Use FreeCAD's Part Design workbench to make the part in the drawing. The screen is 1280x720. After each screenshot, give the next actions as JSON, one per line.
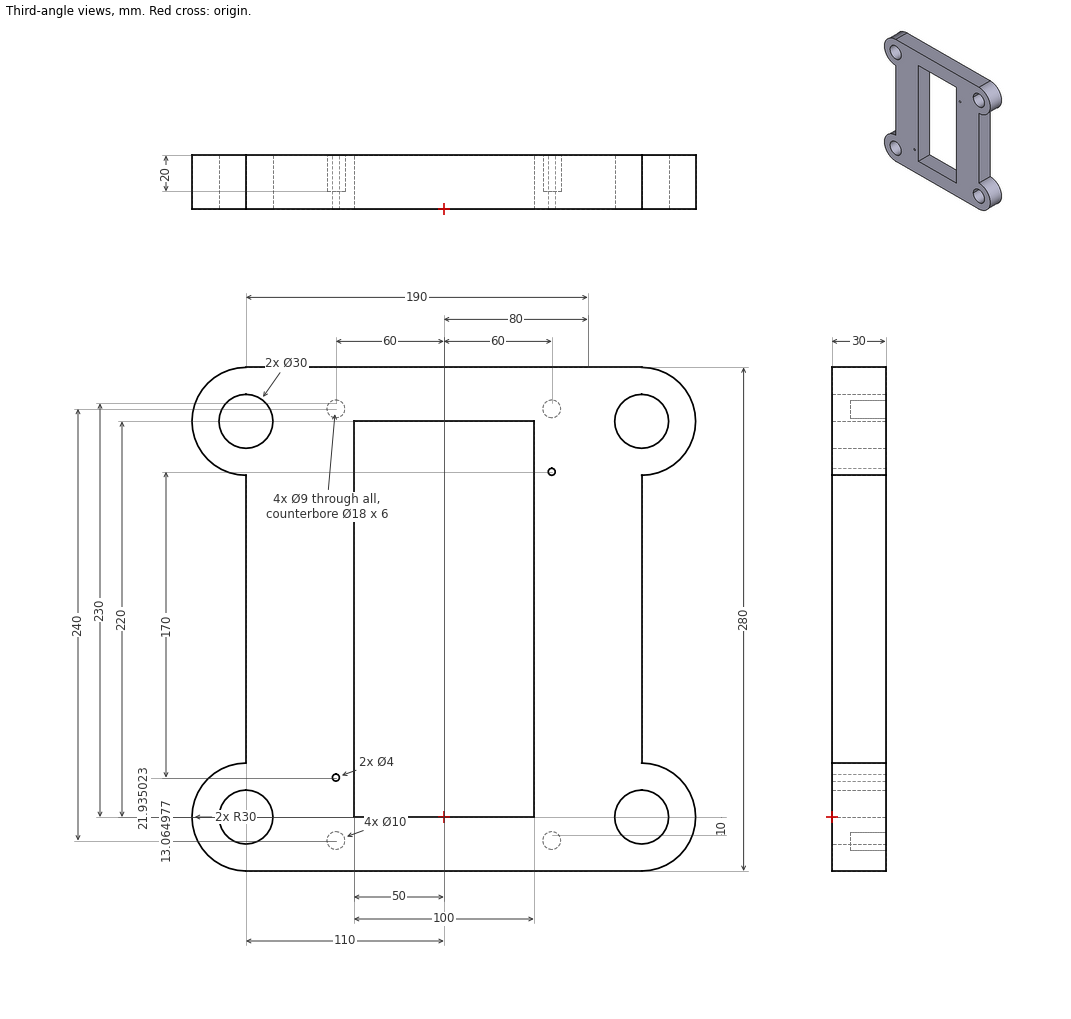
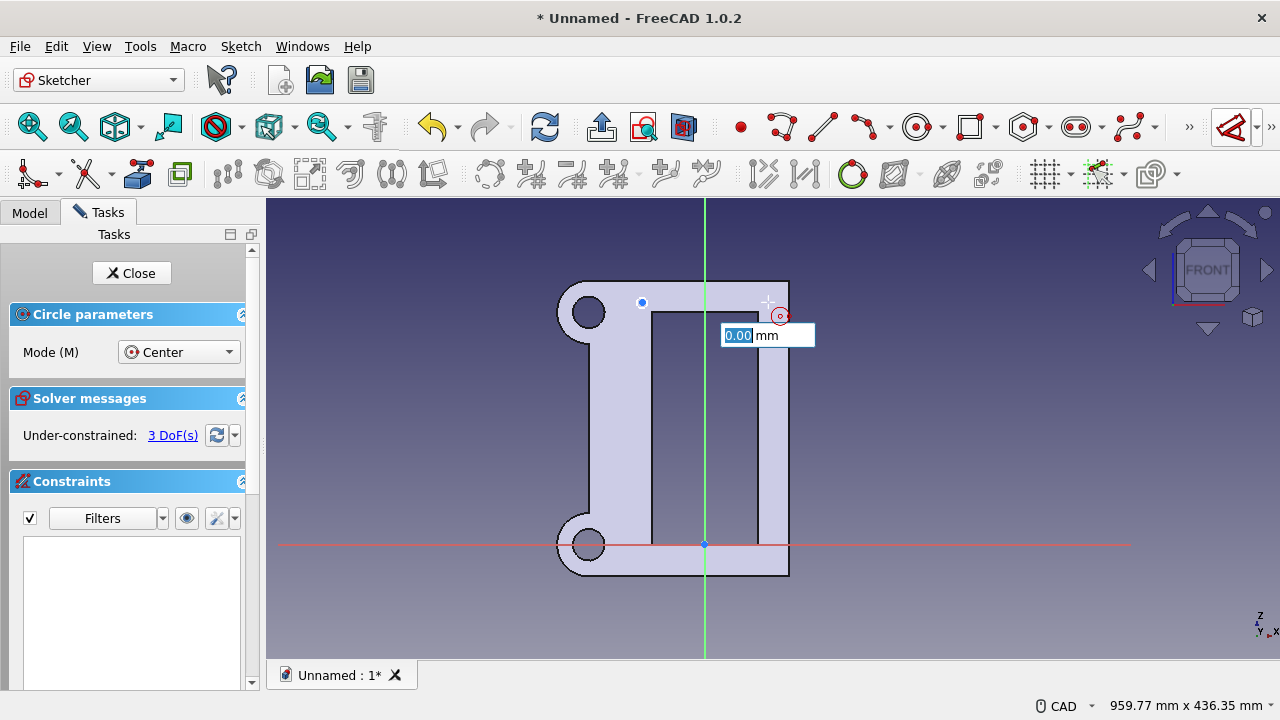
{"action": "scroll", "coordinate": [772, 298], "scroll_direction": "up", "scroll_amount": 7}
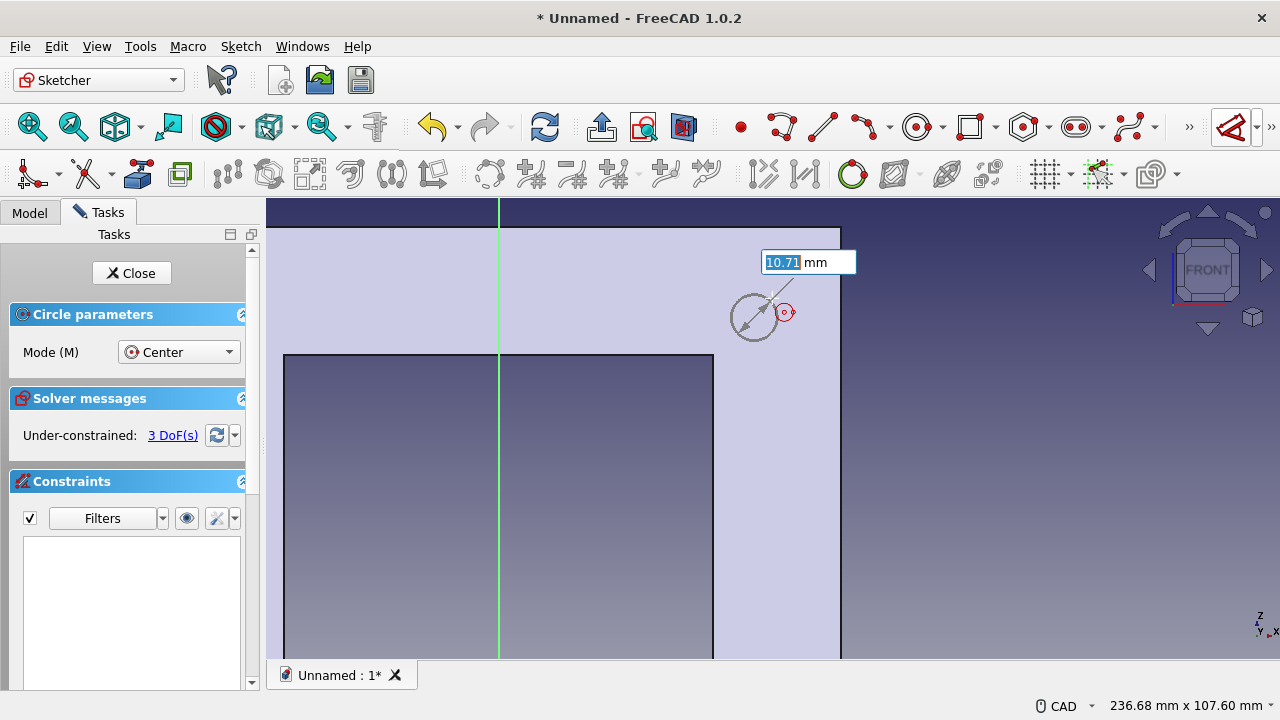
{"action": "left_click", "coordinate": [769, 299]}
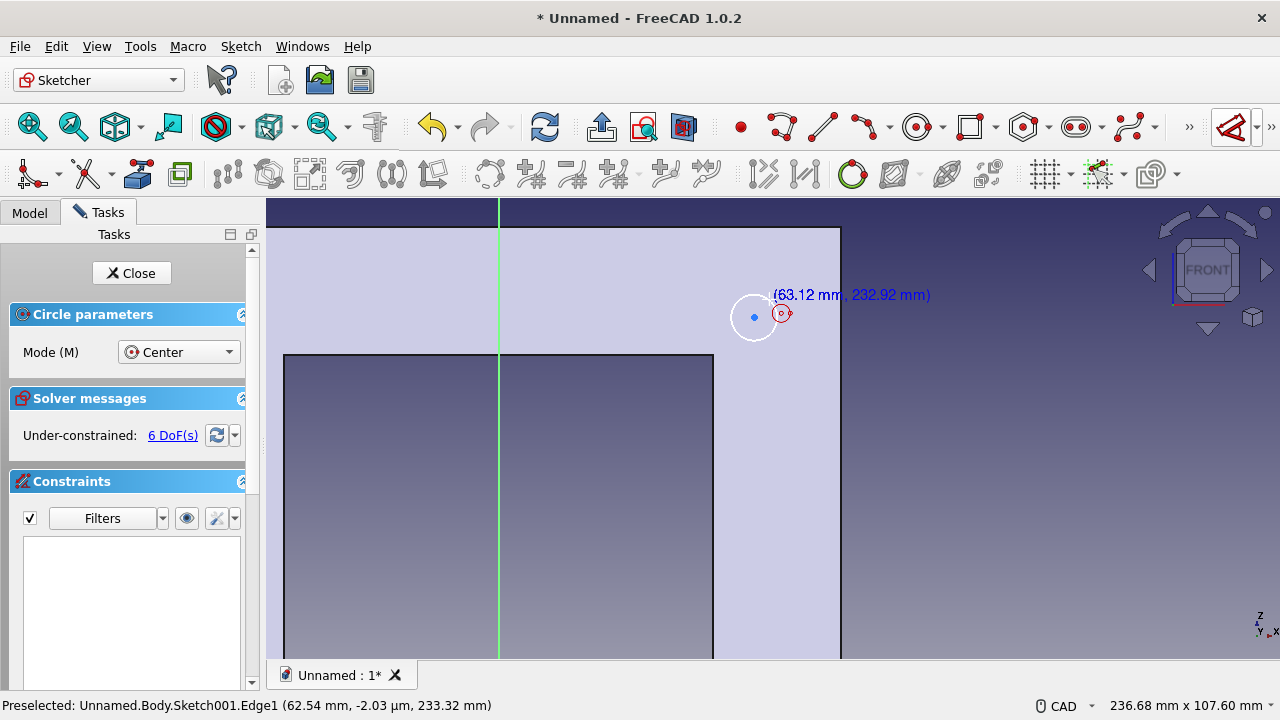
{"action": "scroll", "coordinate": [772, 298], "scroll_direction": "down", "scroll_amount": 7}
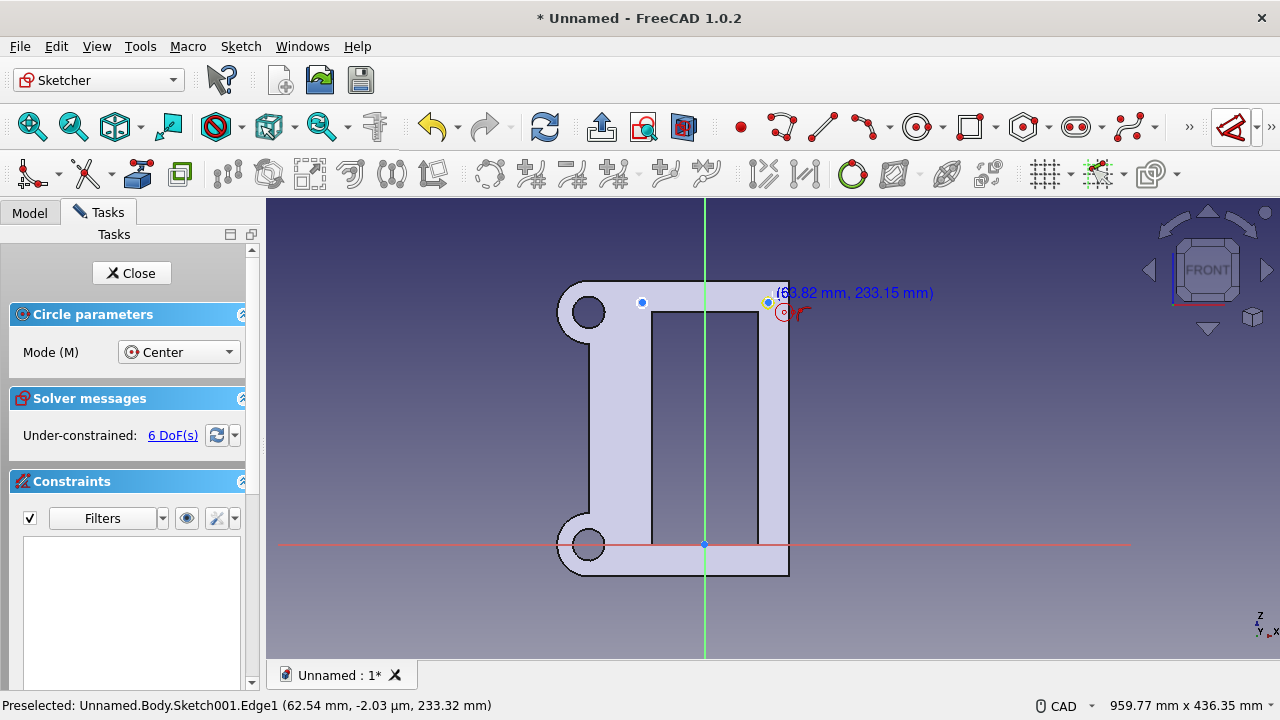
{"action": "scroll", "coordinate": [768, 555], "scroll_direction": "up", "scroll_amount": 8}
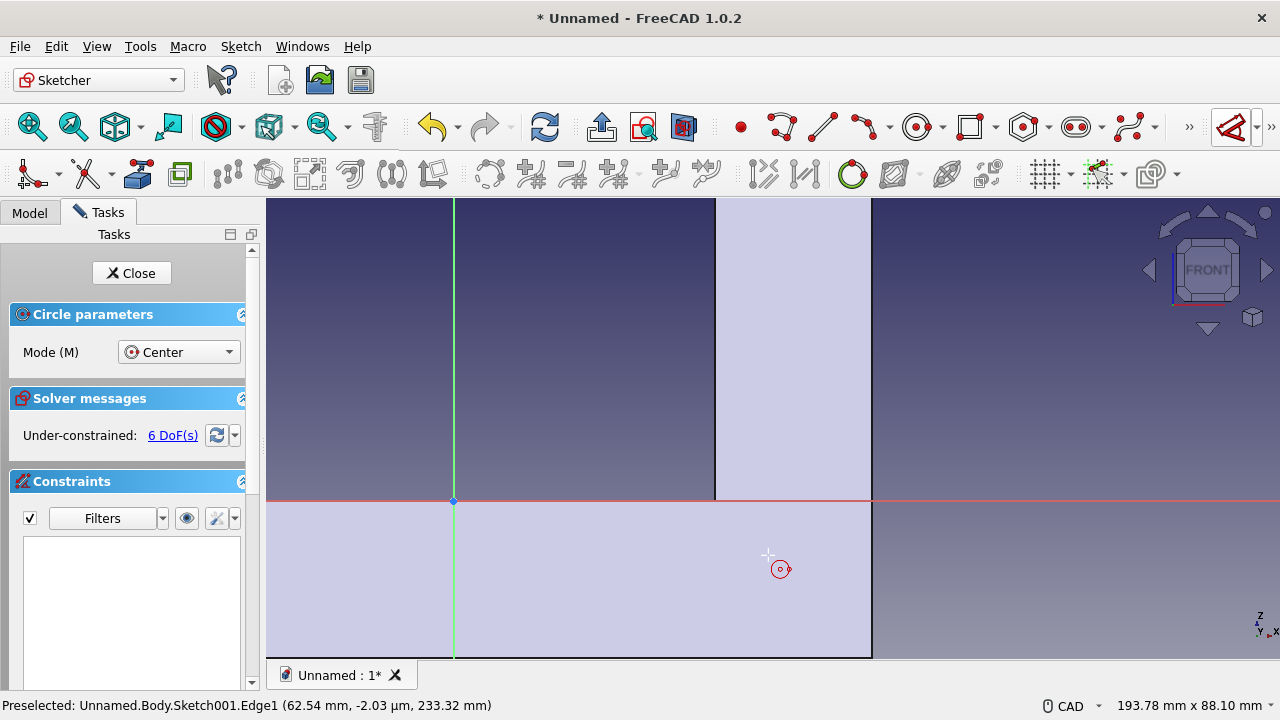
{"action": "scroll", "coordinate": [768, 556], "scroll_direction": "down", "scroll_amount": 8}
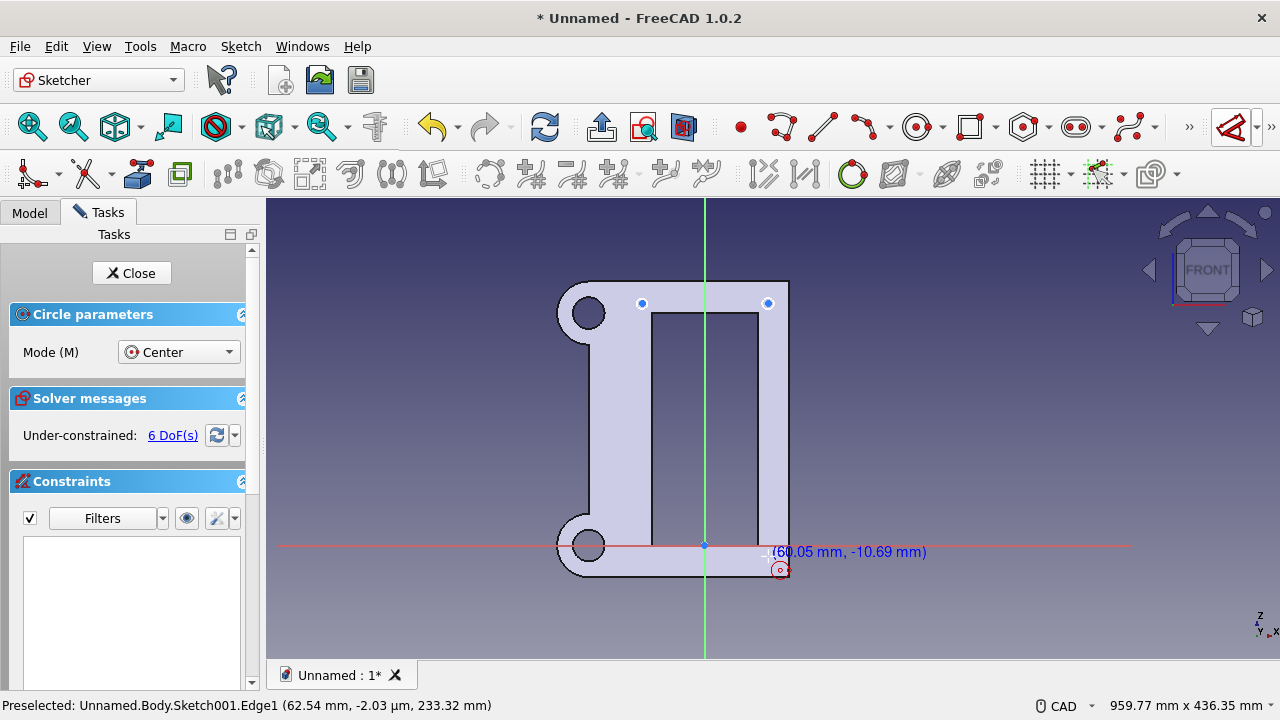
{"action": "scroll", "coordinate": [768, 556], "scroll_direction": "up", "scroll_amount": 3}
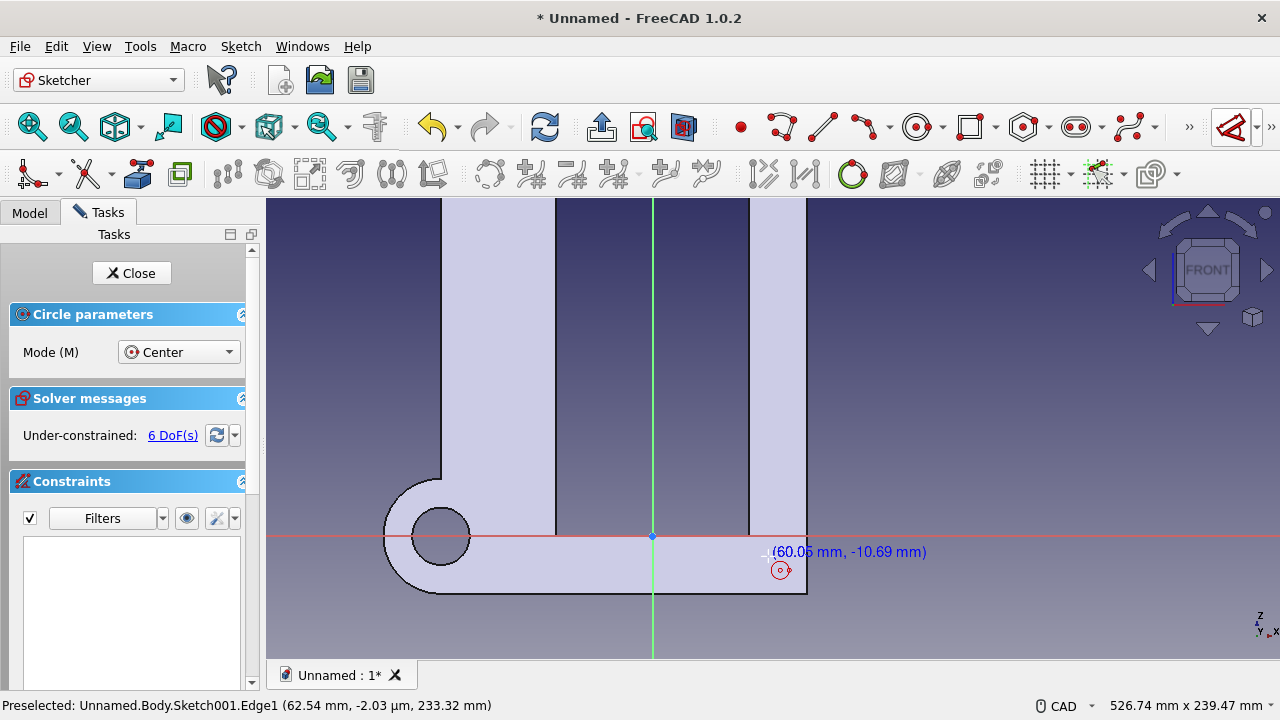
{"action": "left_click", "coordinate": [768, 556]}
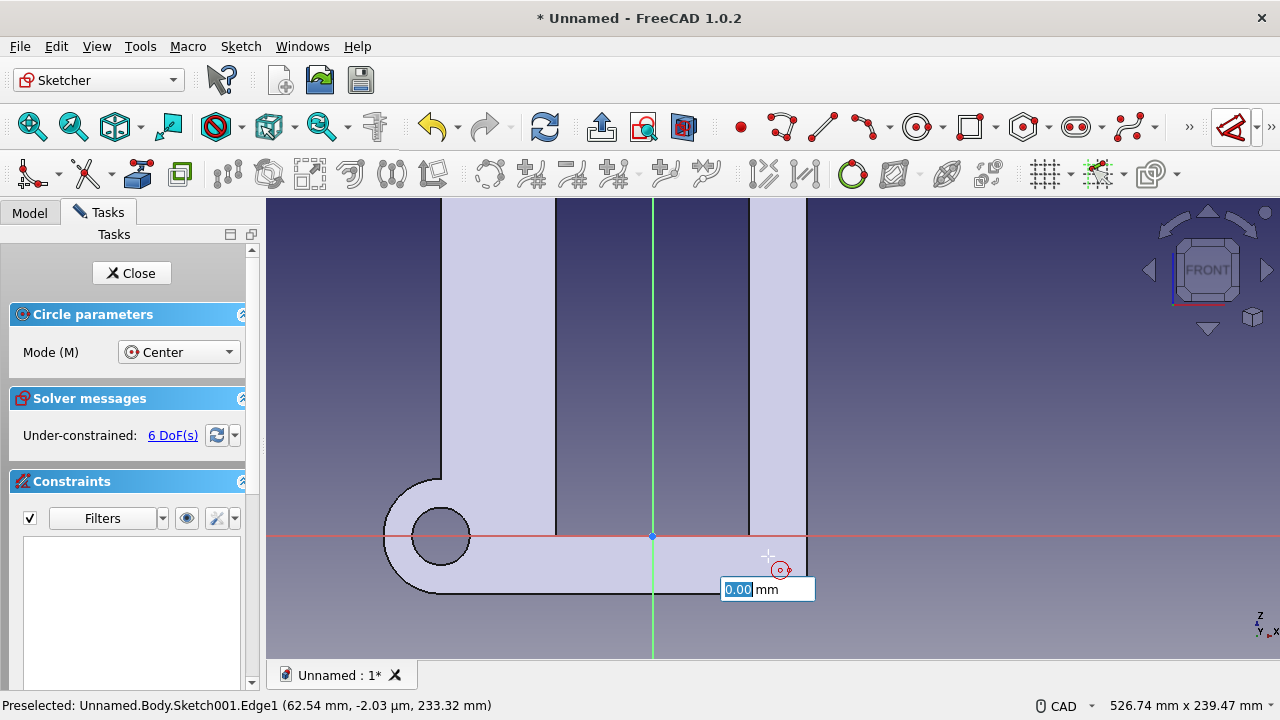
{"action": "scroll", "coordinate": [774, 562], "scroll_direction": "up", "scroll_amount": 4}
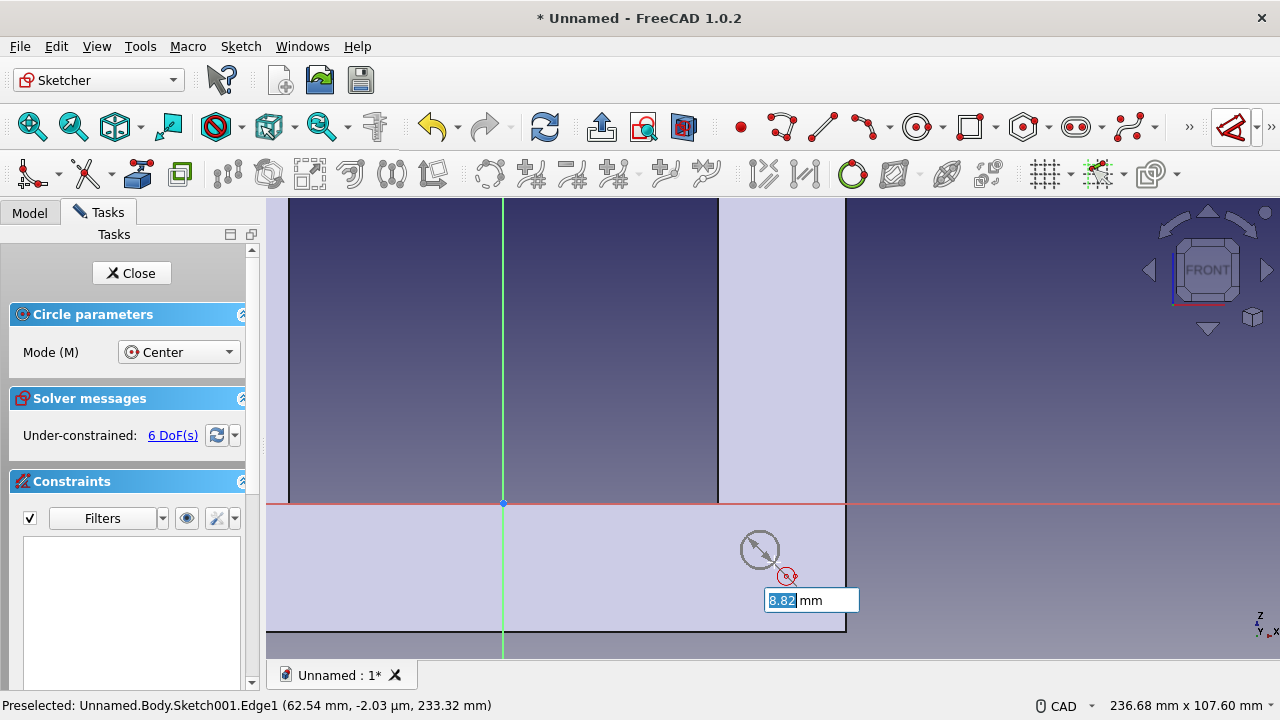
{"action": "left_click", "coordinate": [774, 560]}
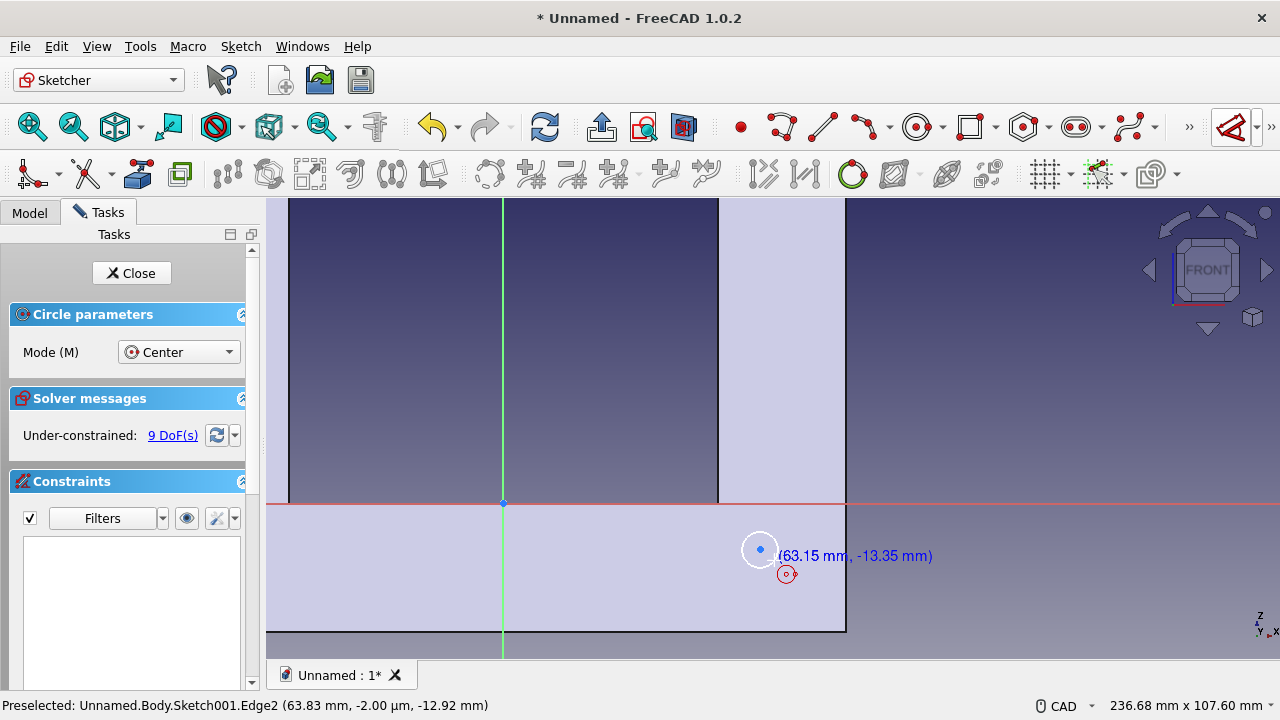
{"action": "scroll", "coordinate": [770, 558], "scroll_direction": "down", "scroll_amount": 7}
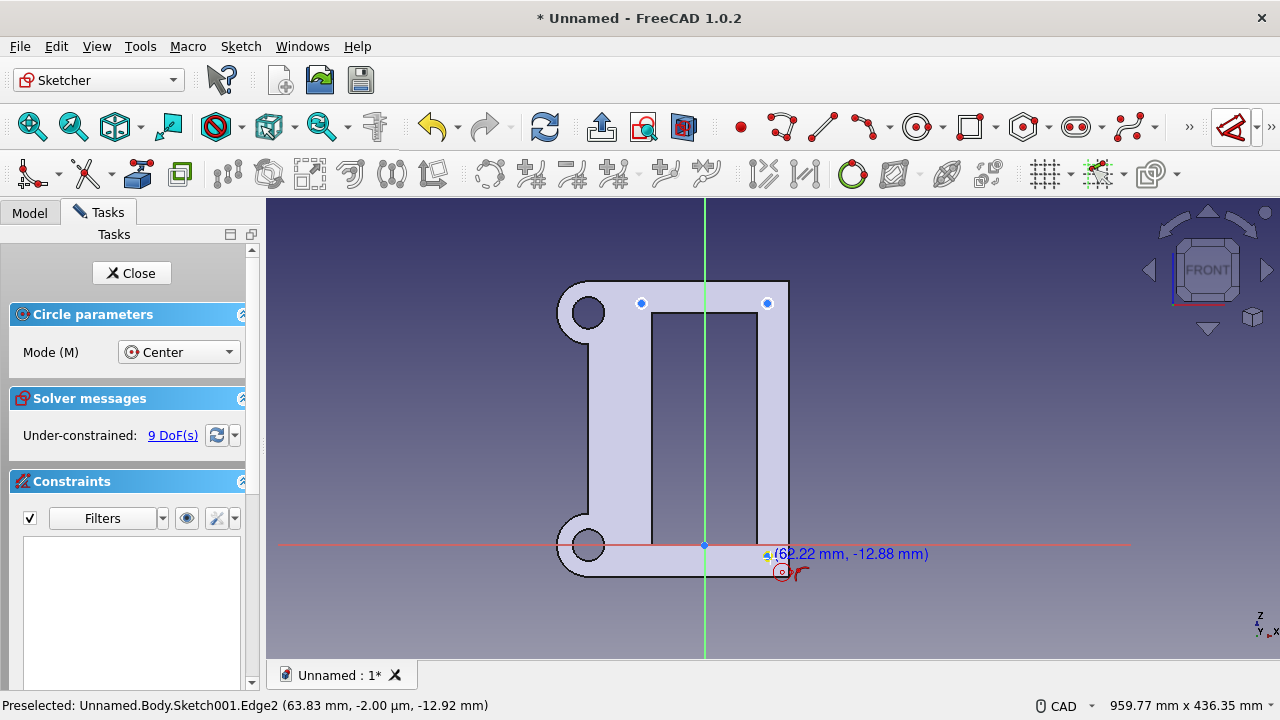
{"action": "scroll", "coordinate": [641, 556], "scroll_direction": "up", "scroll_amount": 8}